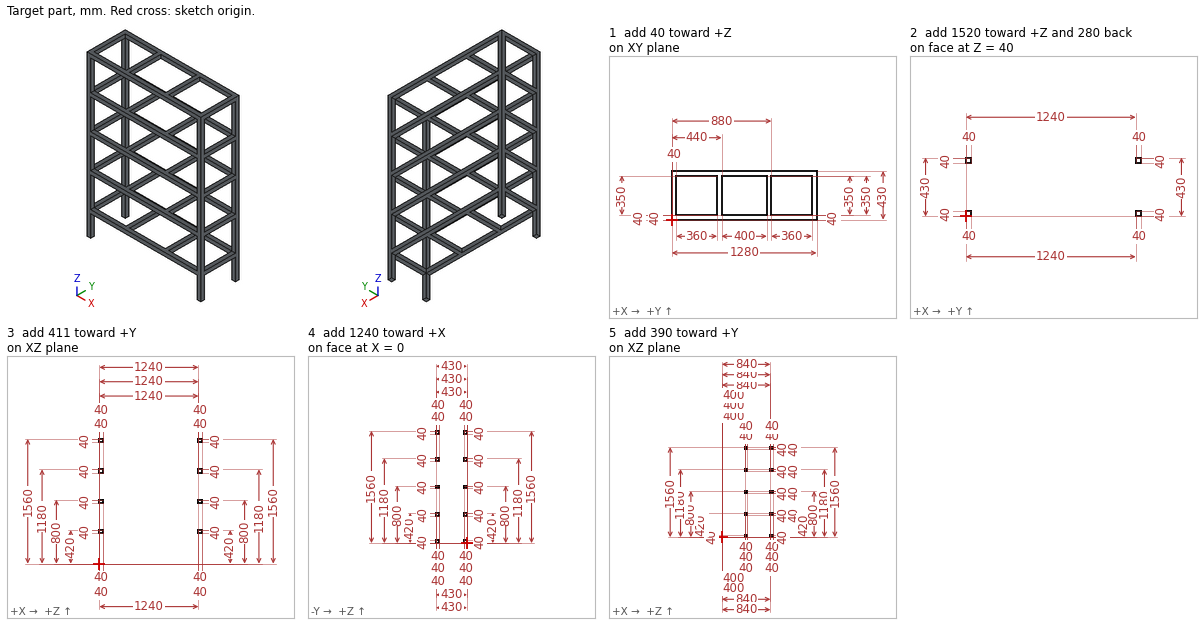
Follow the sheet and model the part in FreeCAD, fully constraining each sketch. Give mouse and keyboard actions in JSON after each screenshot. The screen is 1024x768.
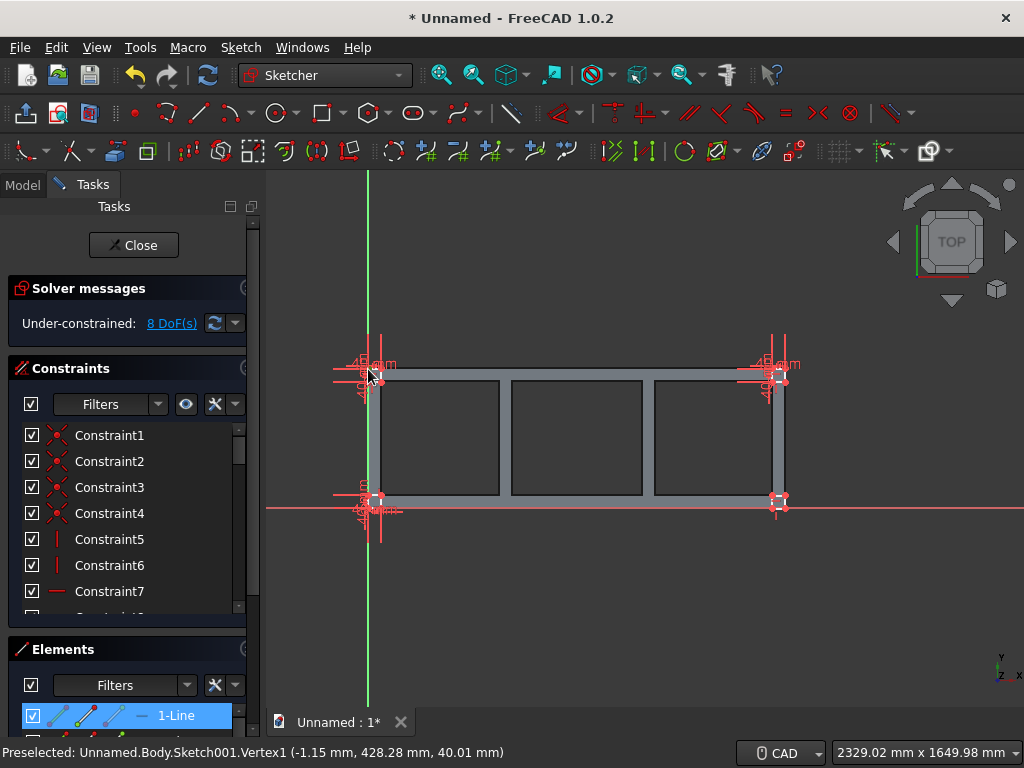
{"action": "left_click", "coordinate": [368, 645]}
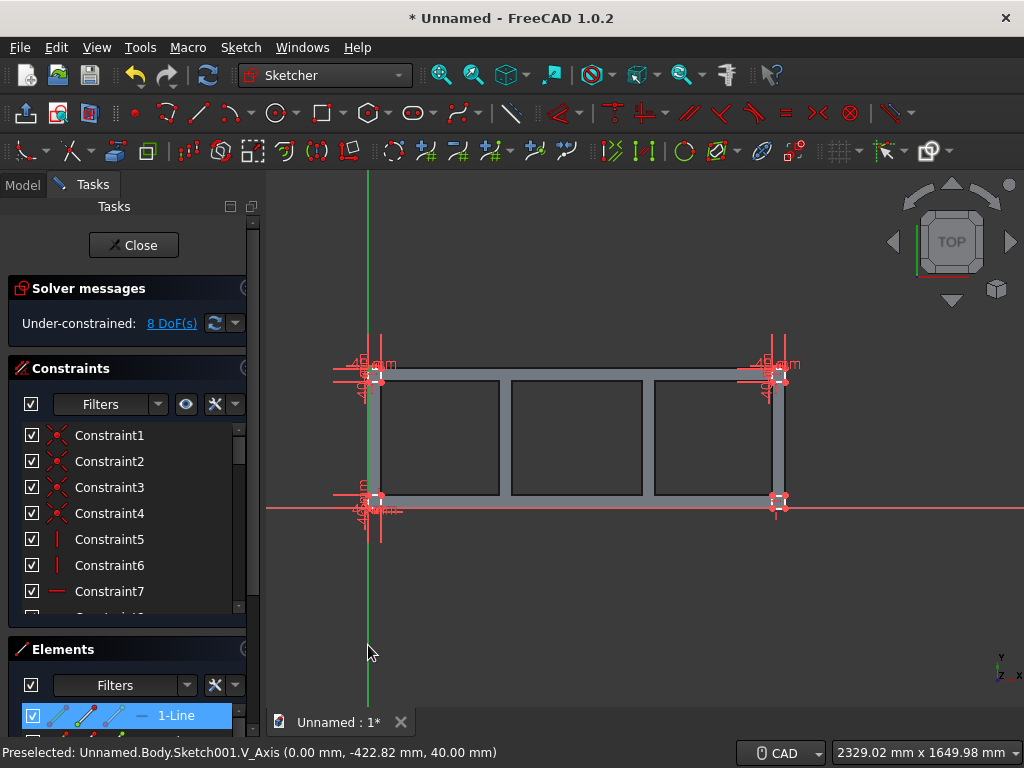
{"action": "left_click", "coordinate": [614, 114]}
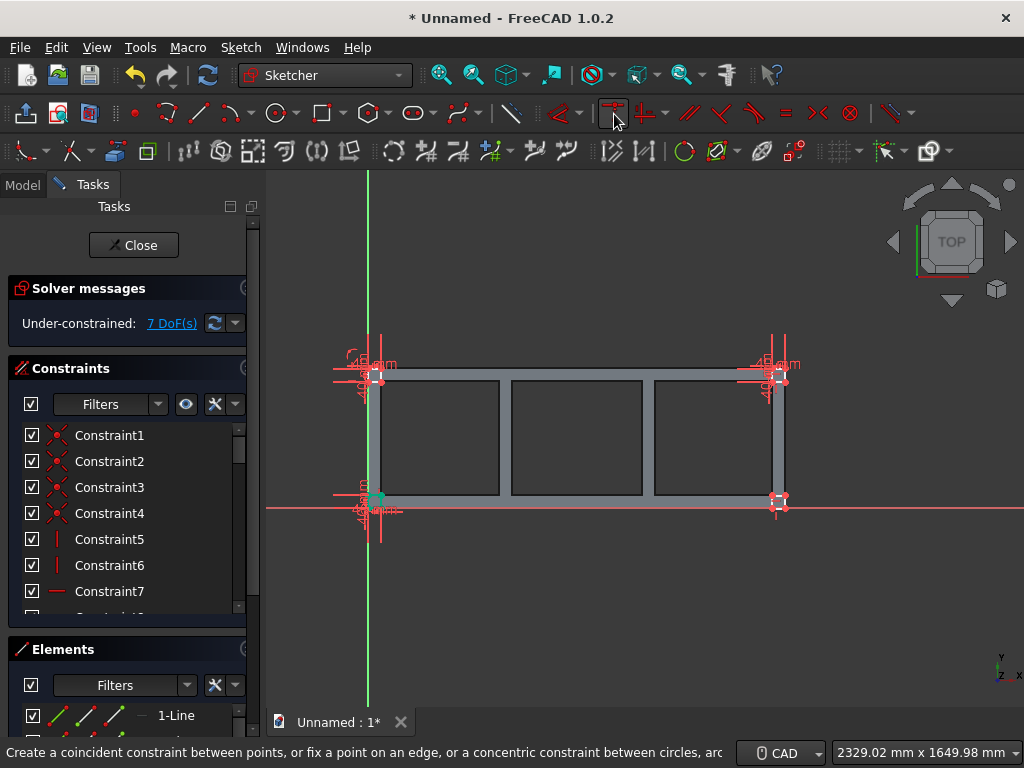
{"action": "left_click", "coordinate": [772, 509]}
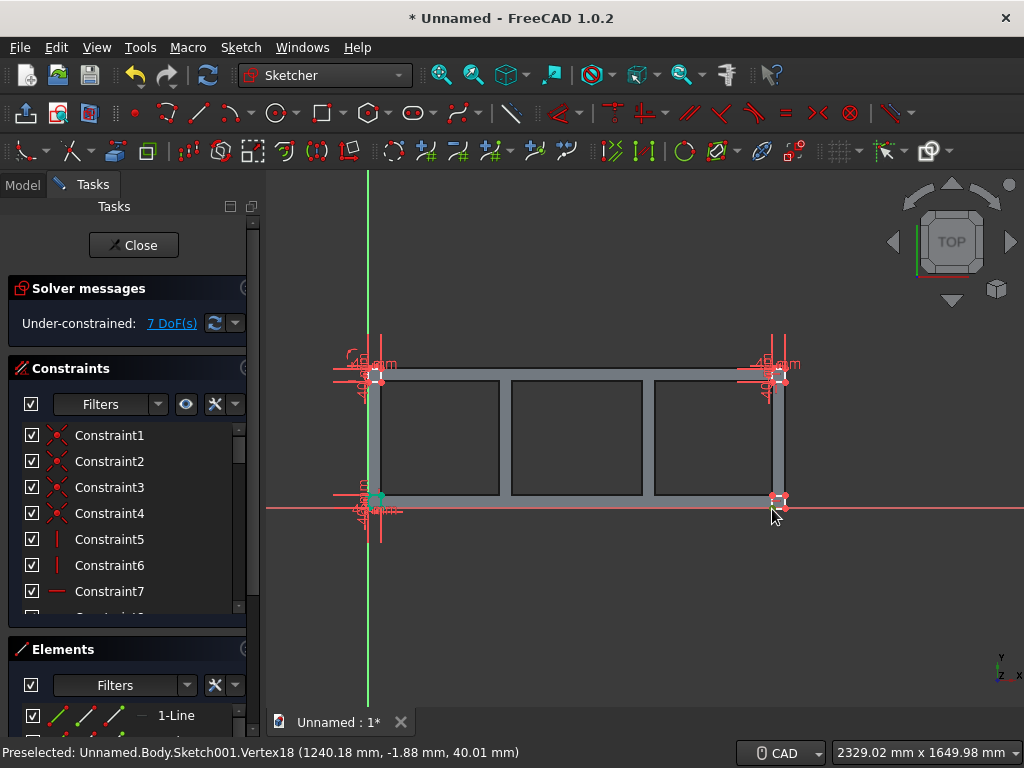
{"action": "left_click", "coordinate": [334, 508]}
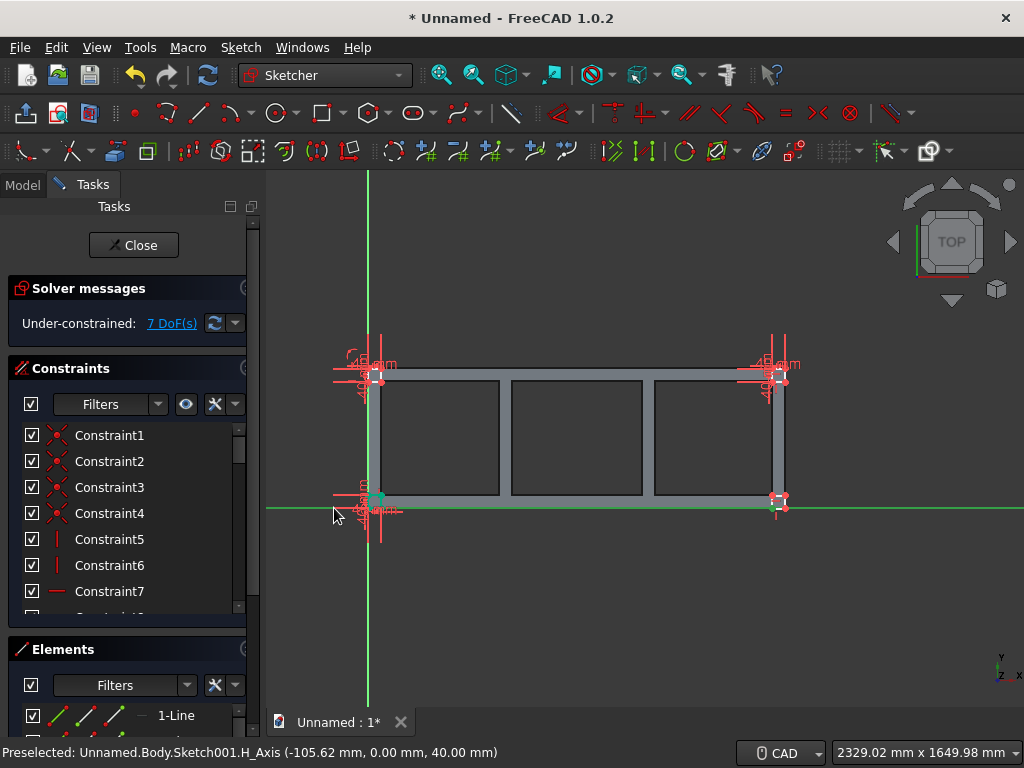
{"action": "left_click", "coordinate": [614, 114]}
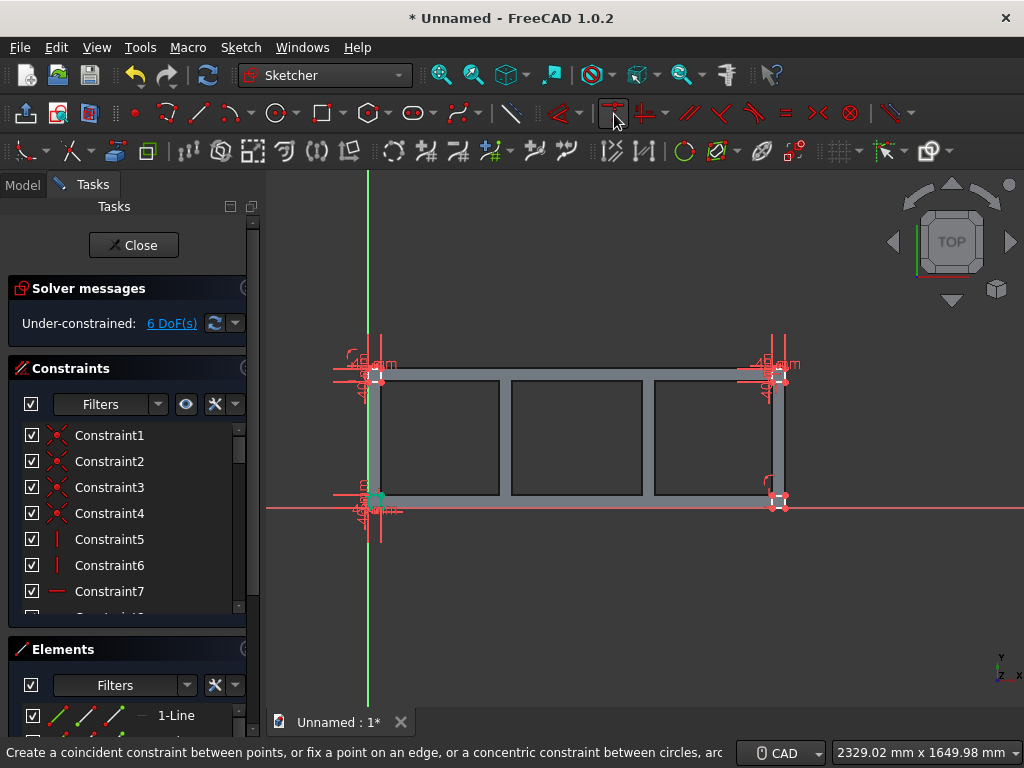
{"action": "left_click", "coordinate": [558, 114]}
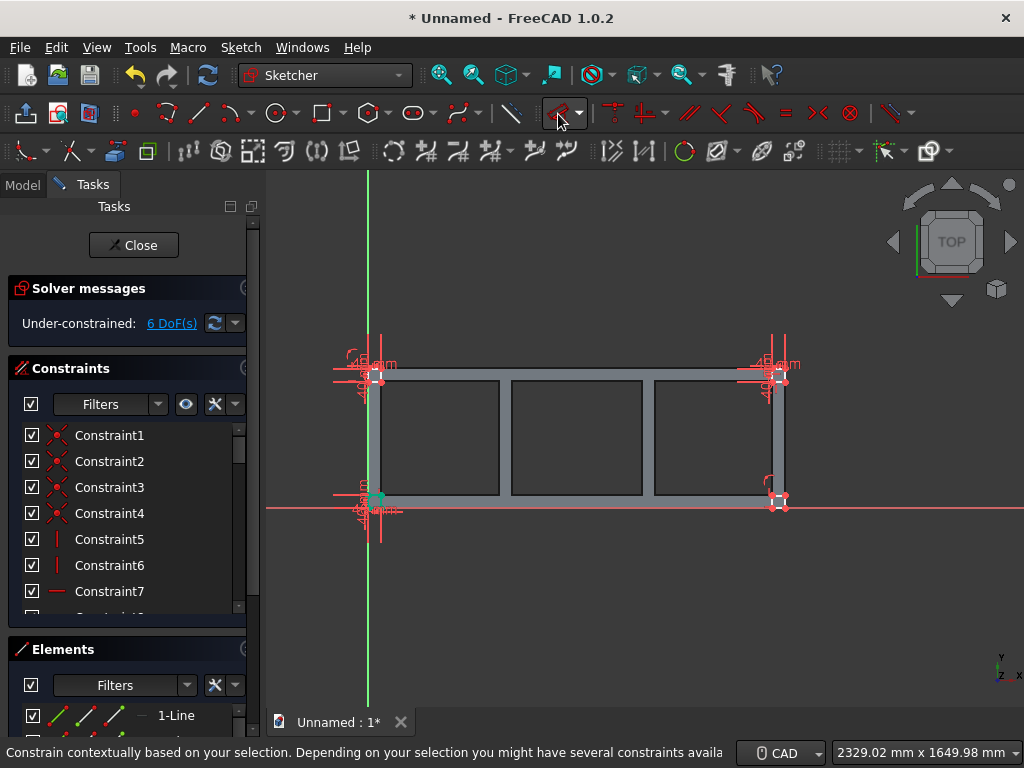
{"action": "scroll", "coordinate": [772, 502], "scroll_direction": "up", "scroll_amount": 6}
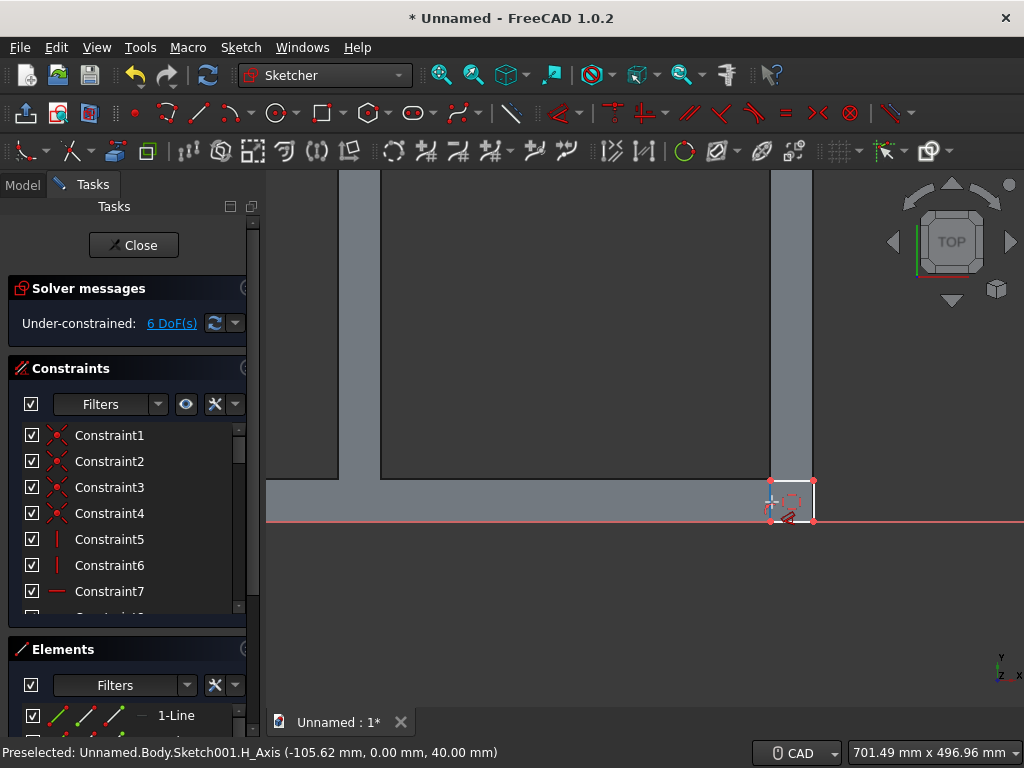
{"action": "left_click", "coordinate": [770, 501]}
{"action": "left_click", "coordinate": [736, 501]}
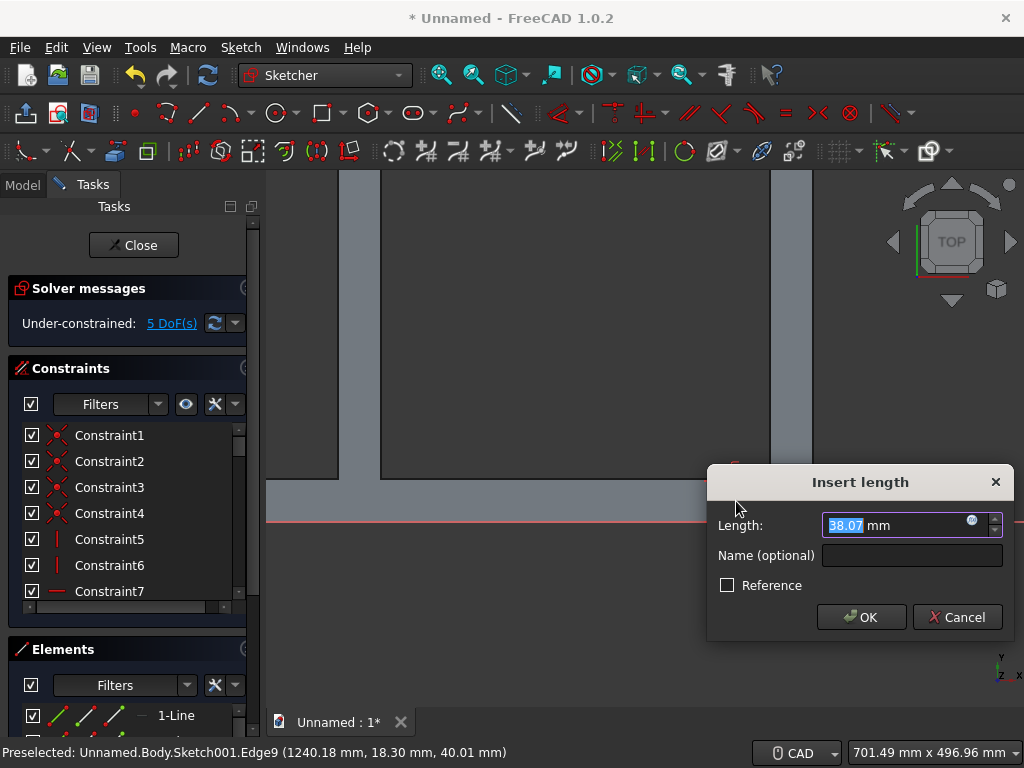
{"action": "type", "text": "40"}
{"action": "key", "text": "Return"}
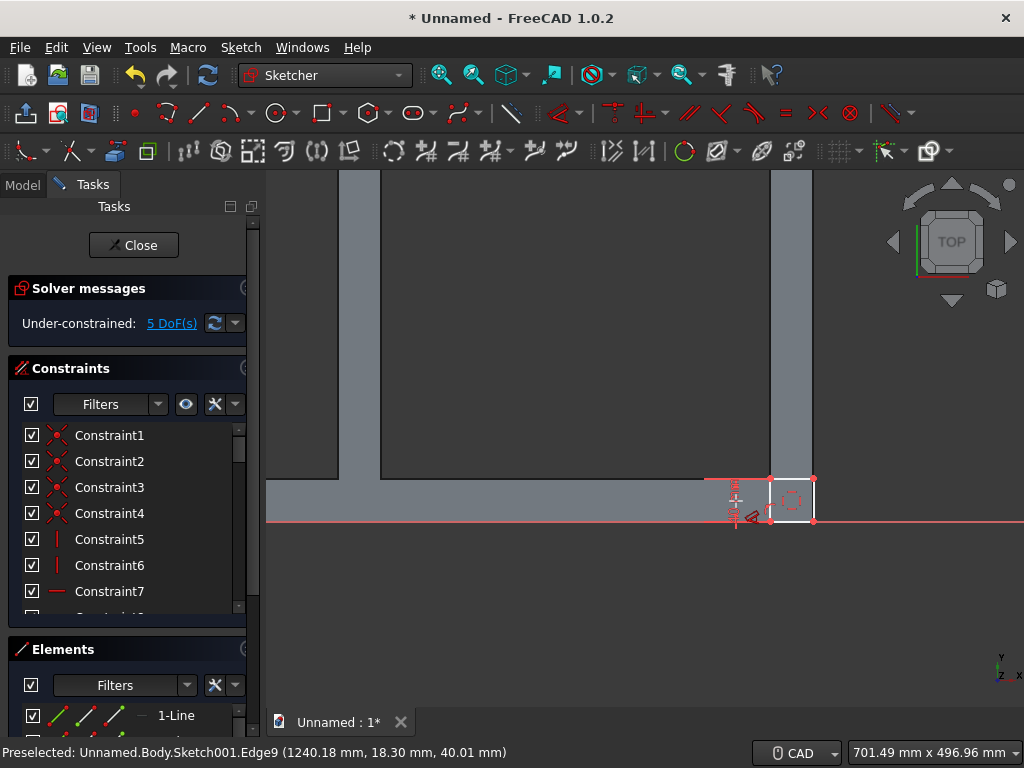
{"action": "left_click", "coordinate": [783, 522]}
{"action": "left_click", "coordinate": [792, 556]}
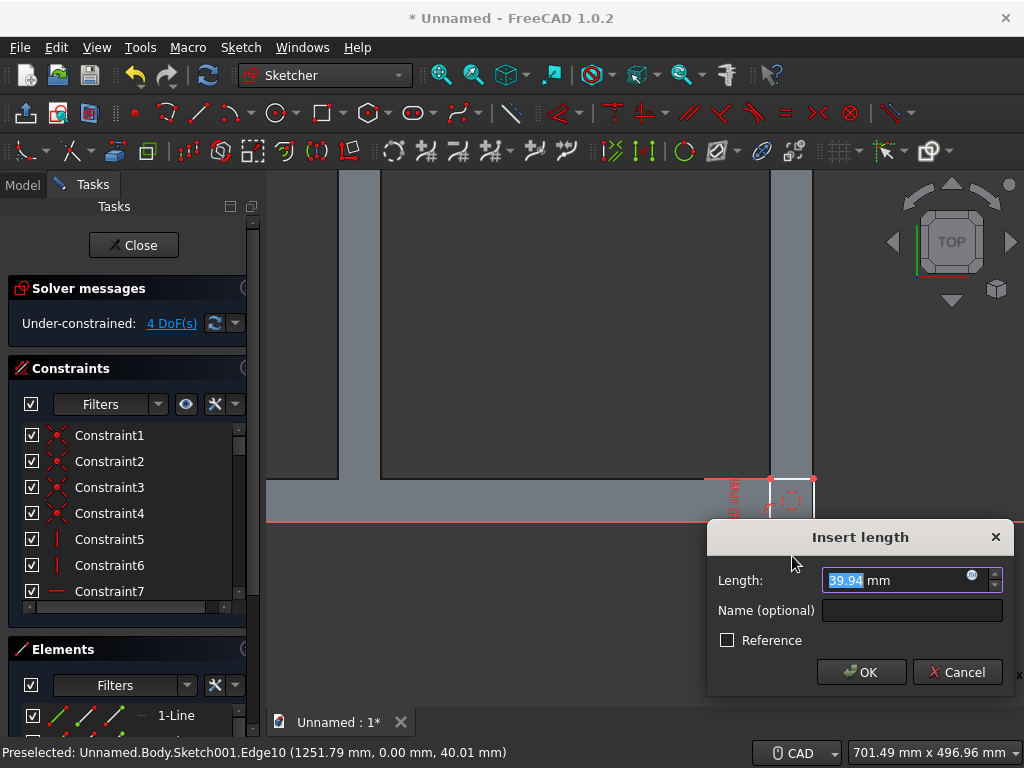
{"action": "type", "text": "40"}
{"action": "key", "text": "Return"}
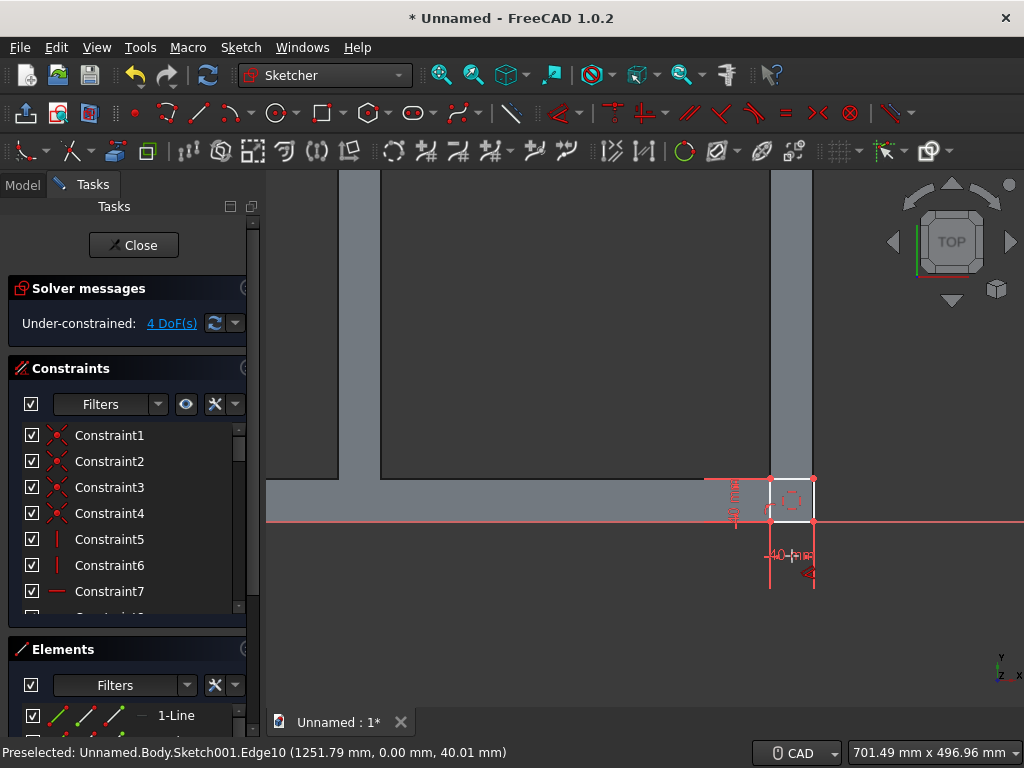
{"action": "scroll", "coordinate": [772, 503], "scroll_direction": "down", "scroll_amount": 6}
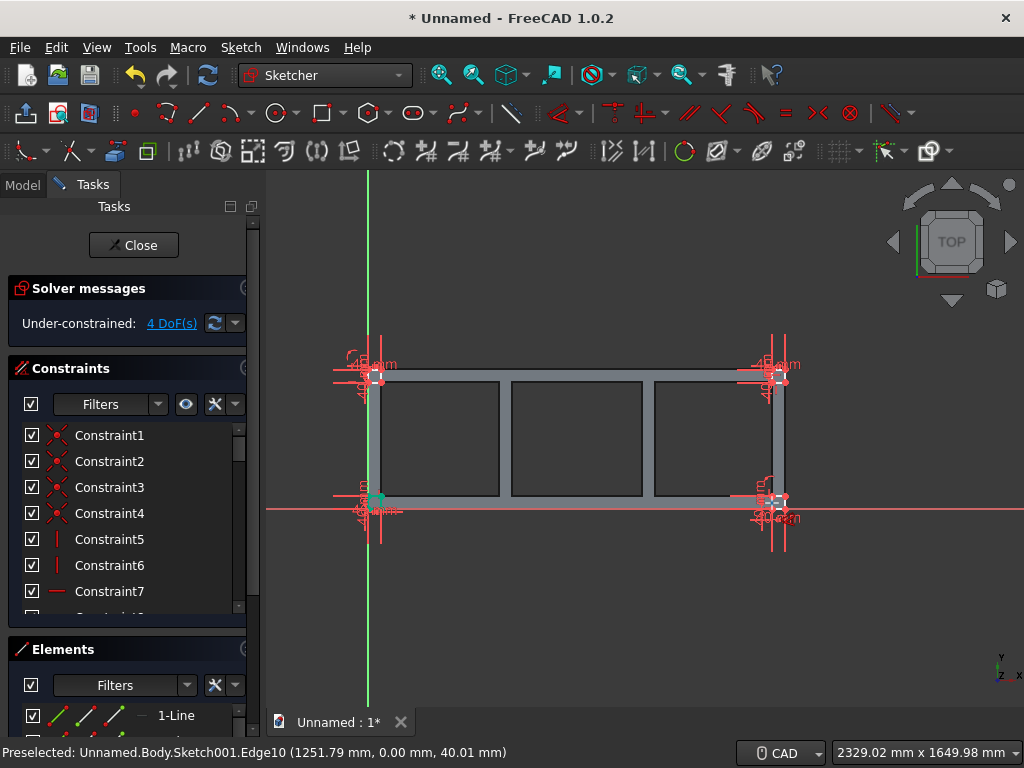
{"action": "left_click", "coordinate": [368, 370]}
{"action": "left_click", "coordinate": [334, 439]}